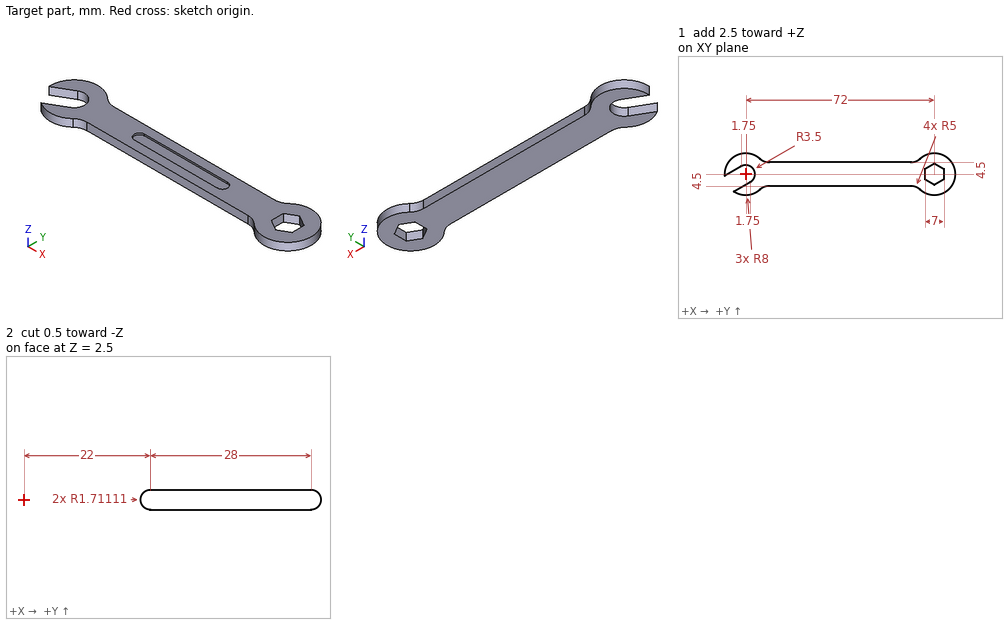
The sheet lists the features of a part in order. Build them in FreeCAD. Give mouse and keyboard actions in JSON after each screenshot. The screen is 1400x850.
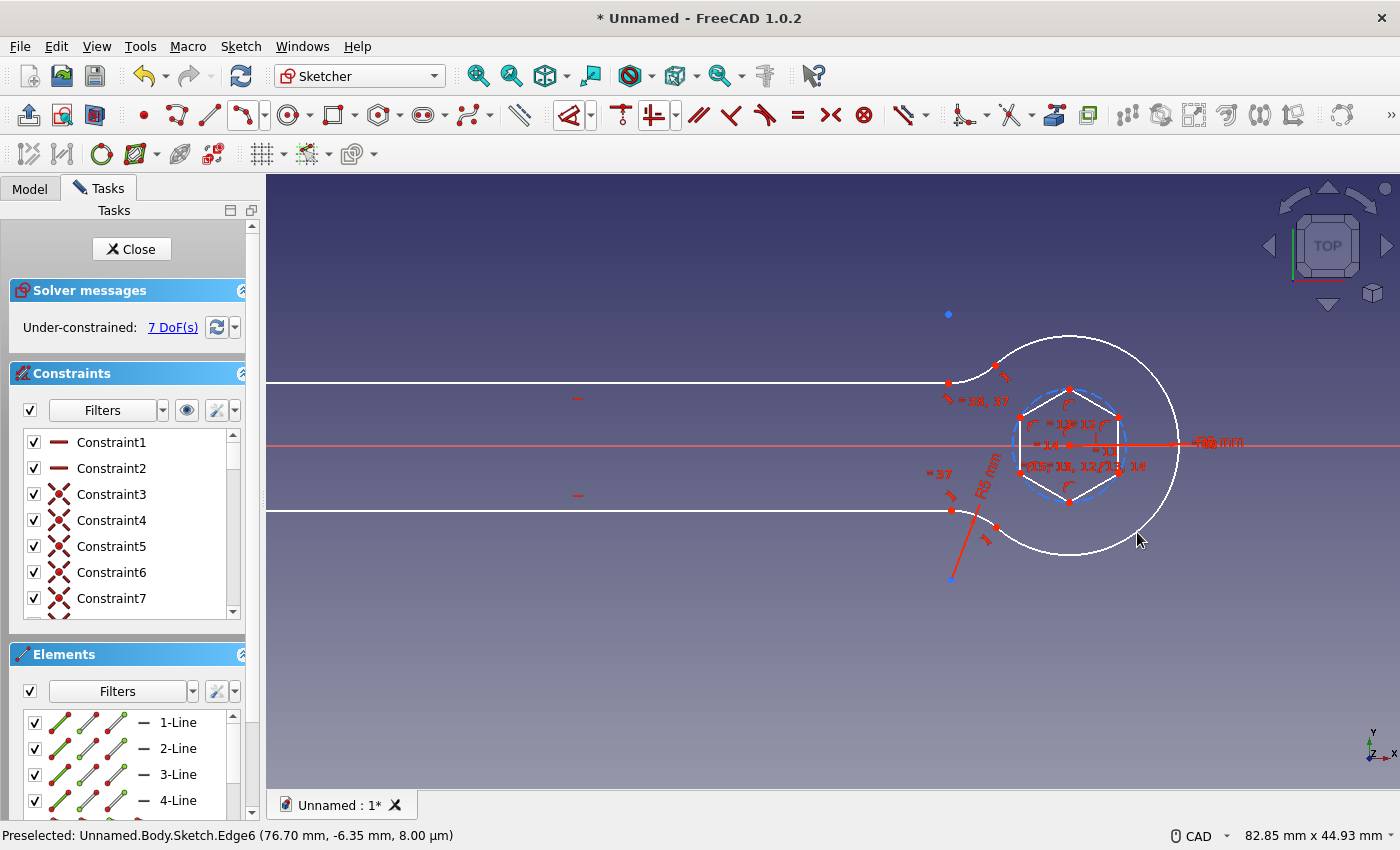
{"action": "scroll", "coordinate": [989, 519], "scroll_direction": "down", "scroll_amount": 3}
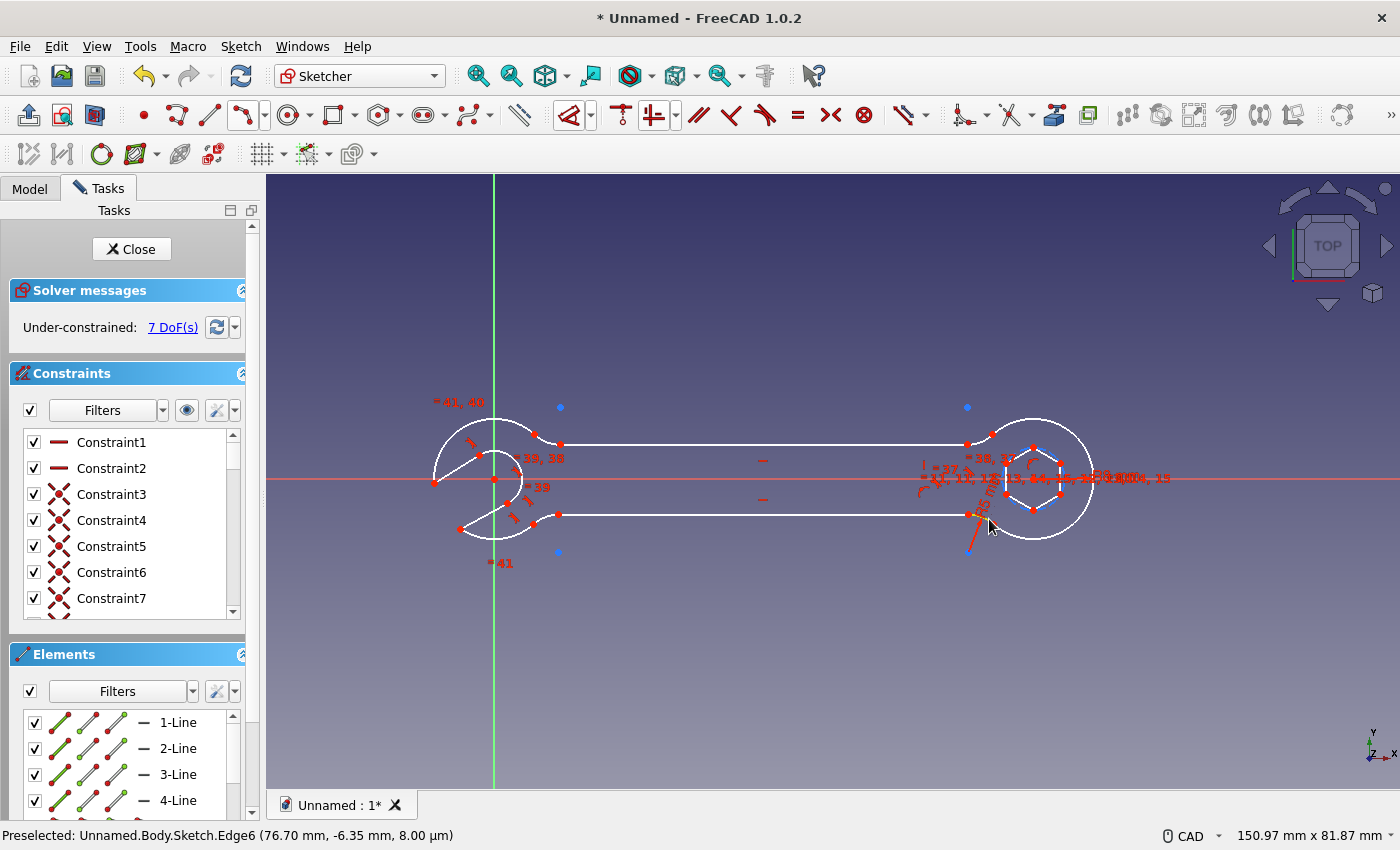
{"action": "scroll", "coordinate": [505, 453], "scroll_direction": "up", "scroll_amount": 3}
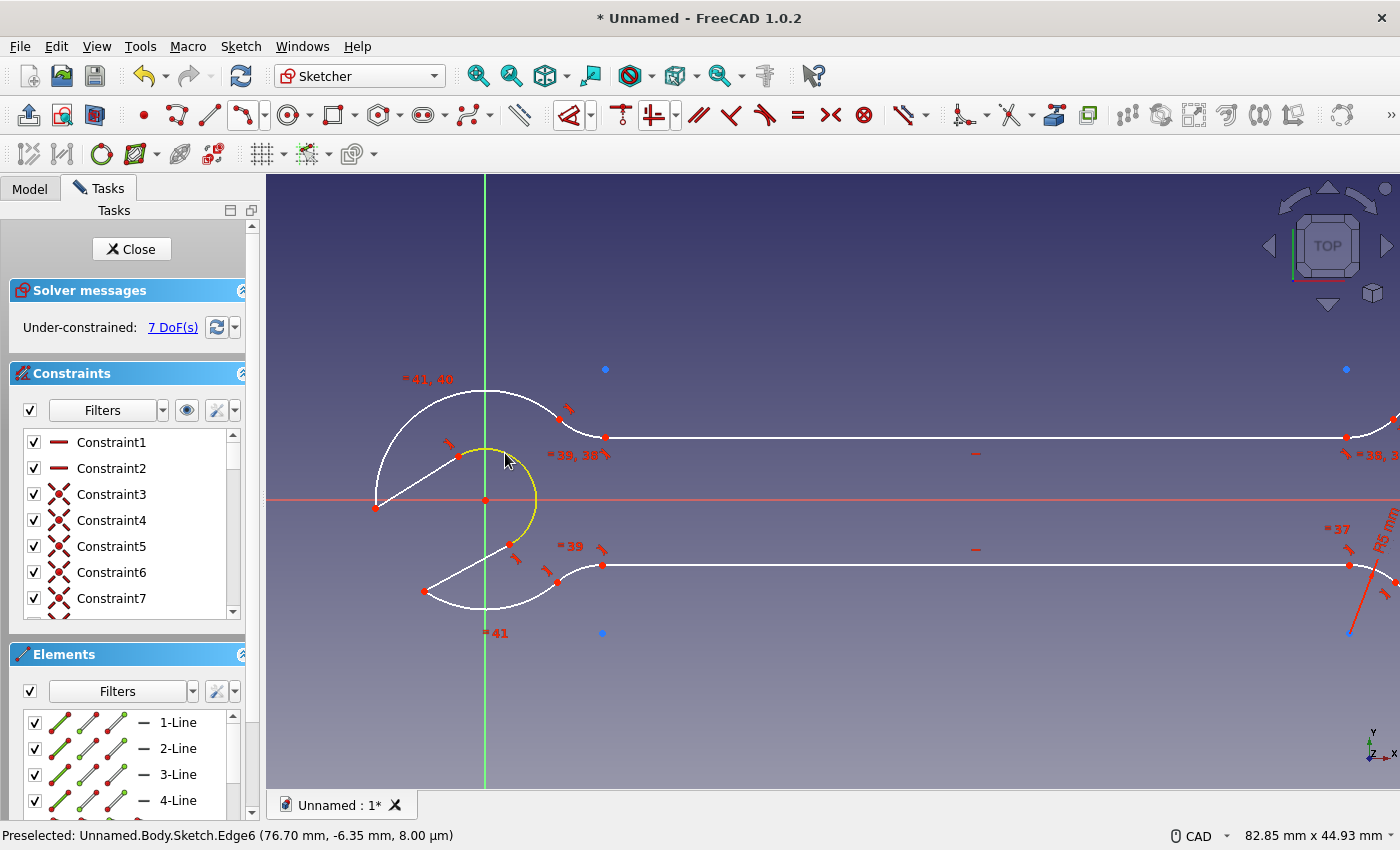
{"action": "left_click", "coordinate": [505, 453]}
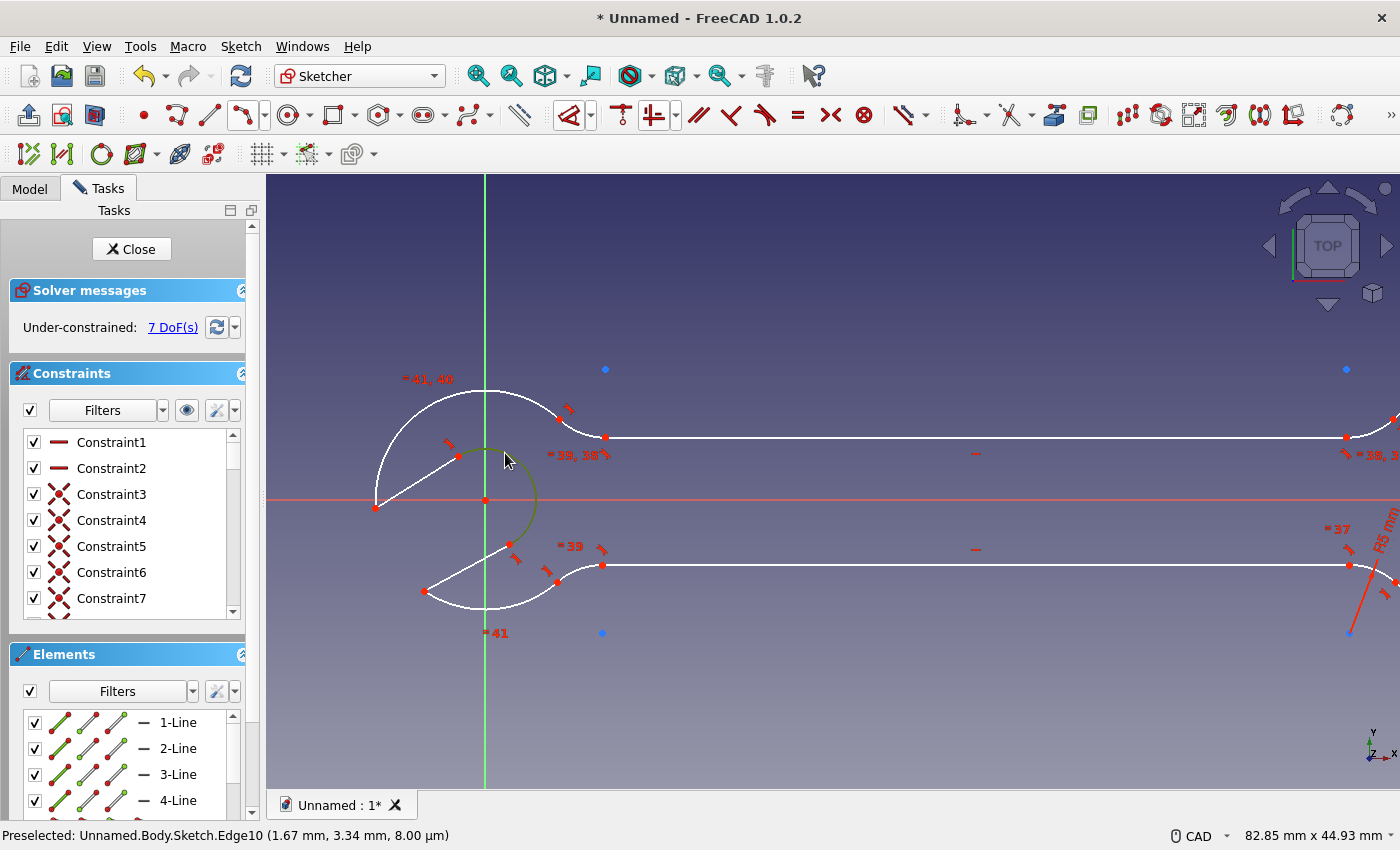
{"action": "key", "text": "k r"}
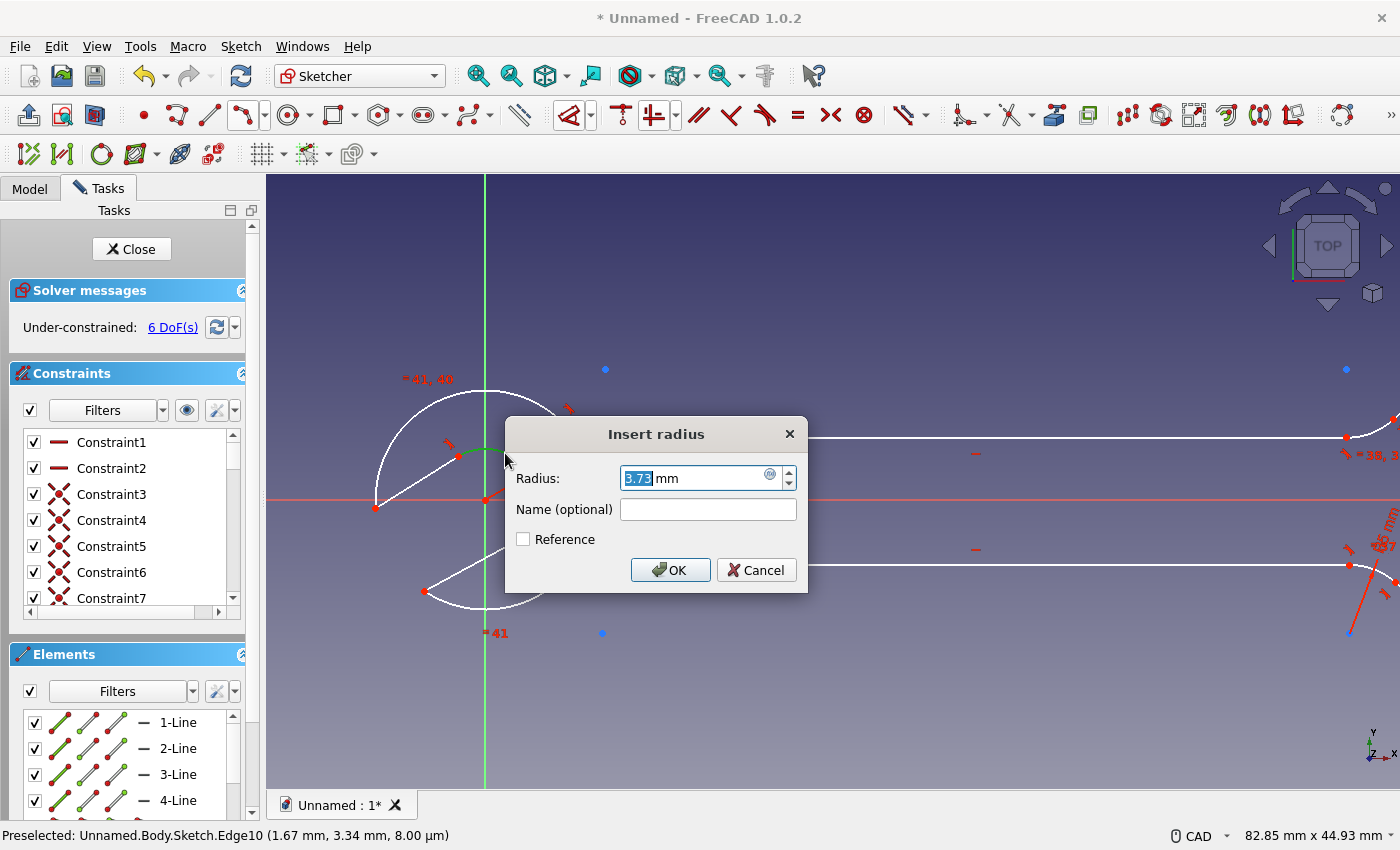
{"action": "type", "text": "3.5"}
{"action": "key", "text": "Return"}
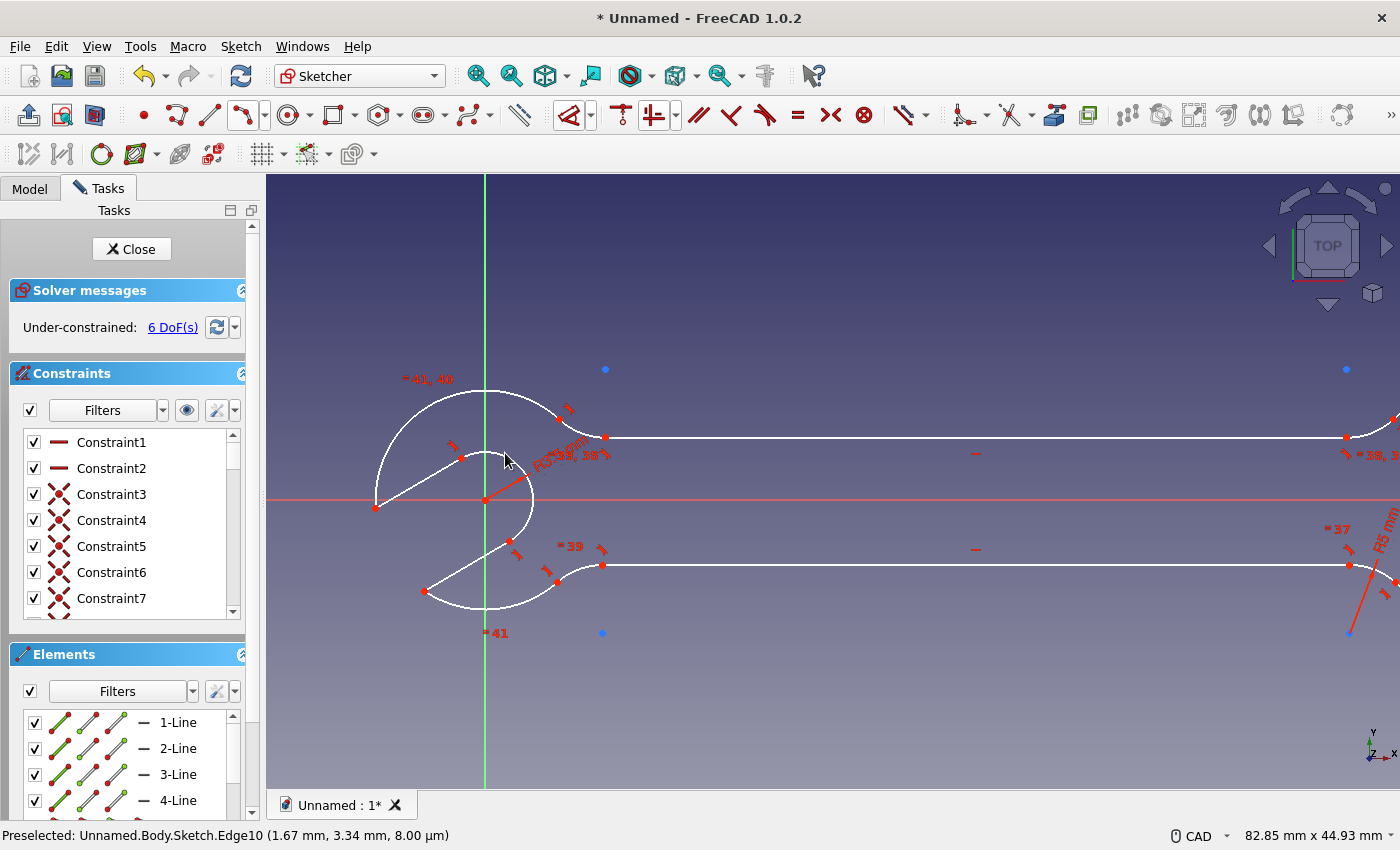
{"action": "scroll", "coordinate": [505, 453], "scroll_direction": "down", "scroll_amount": 3}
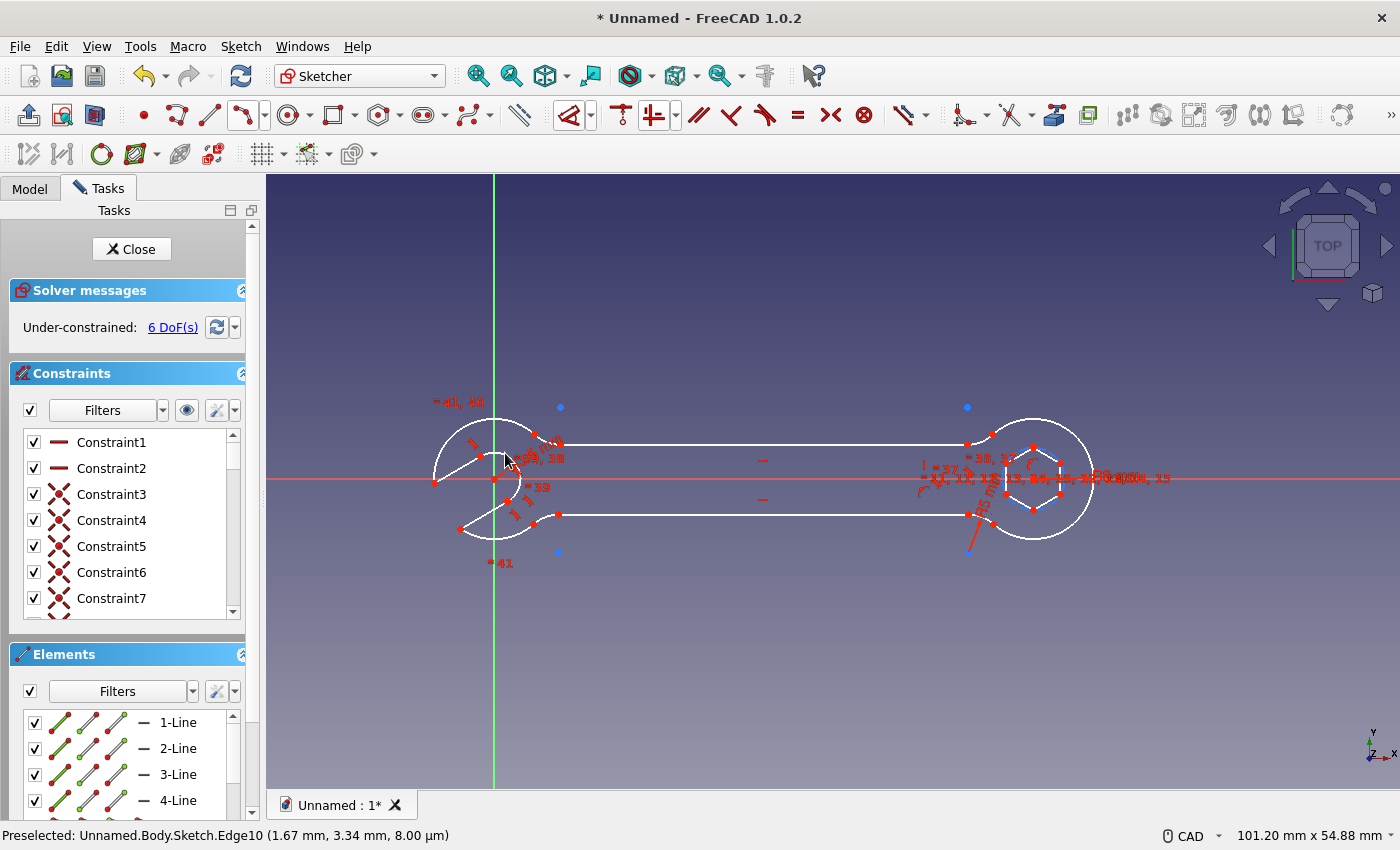
{"action": "left_click", "coordinate": [1006, 463]}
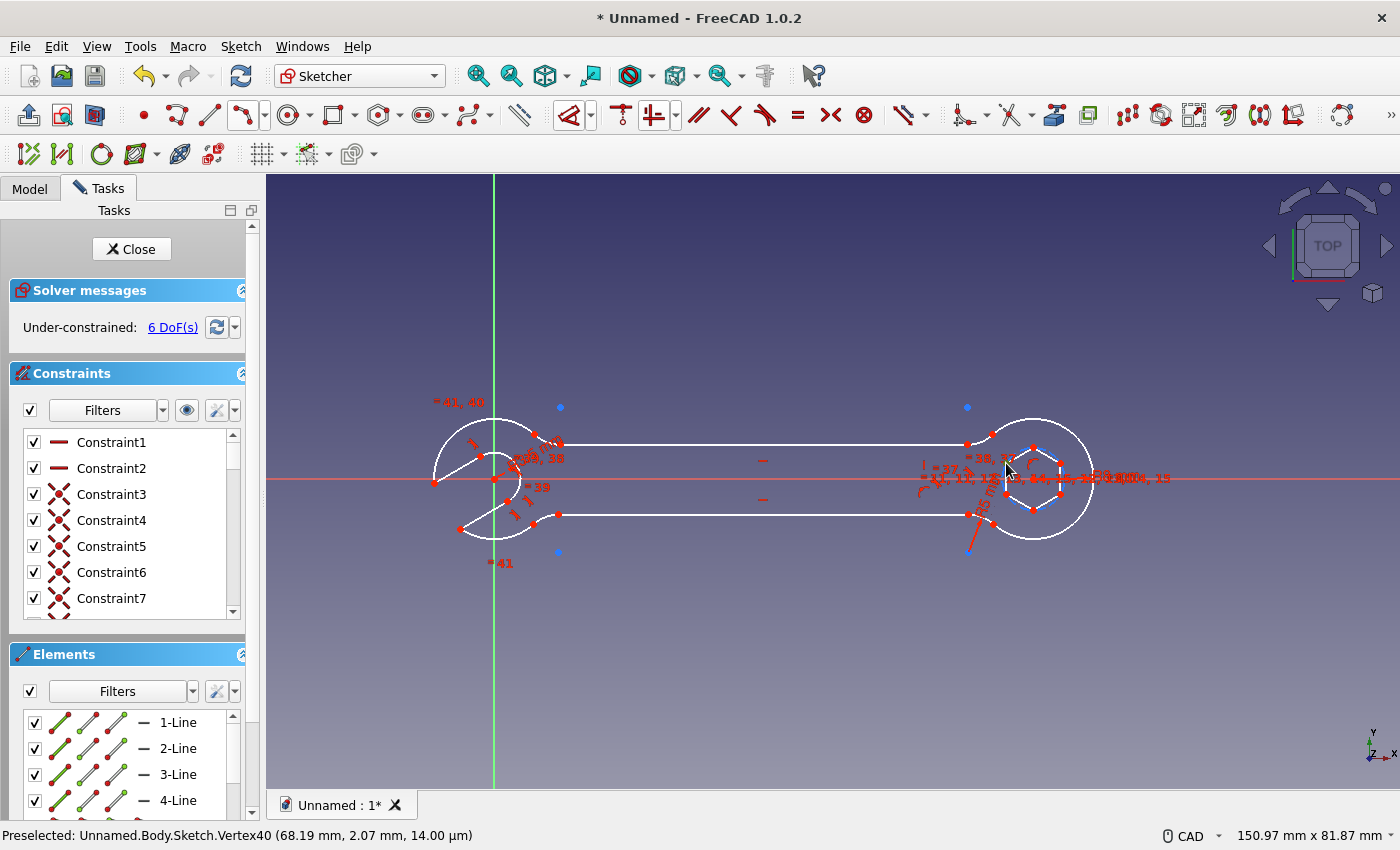
{"action": "left_click", "coordinate": [1060, 495]}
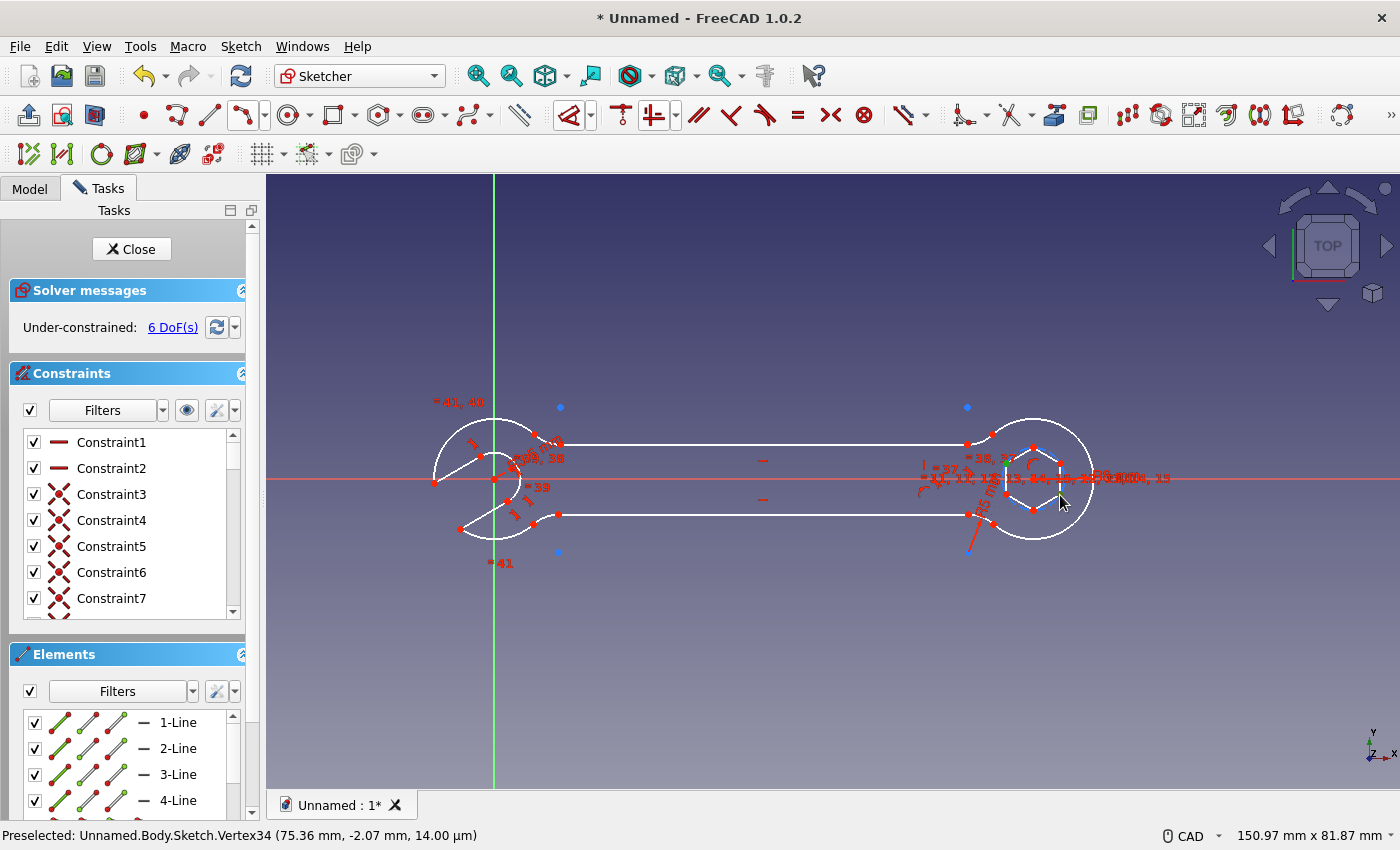
{"action": "key", "text": "l"}